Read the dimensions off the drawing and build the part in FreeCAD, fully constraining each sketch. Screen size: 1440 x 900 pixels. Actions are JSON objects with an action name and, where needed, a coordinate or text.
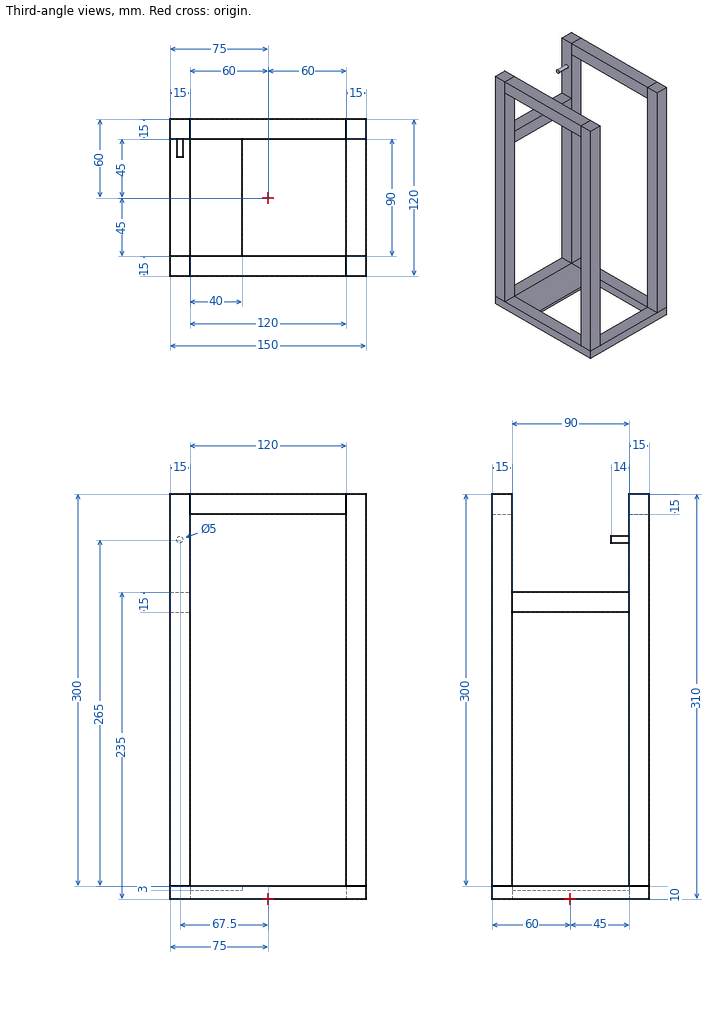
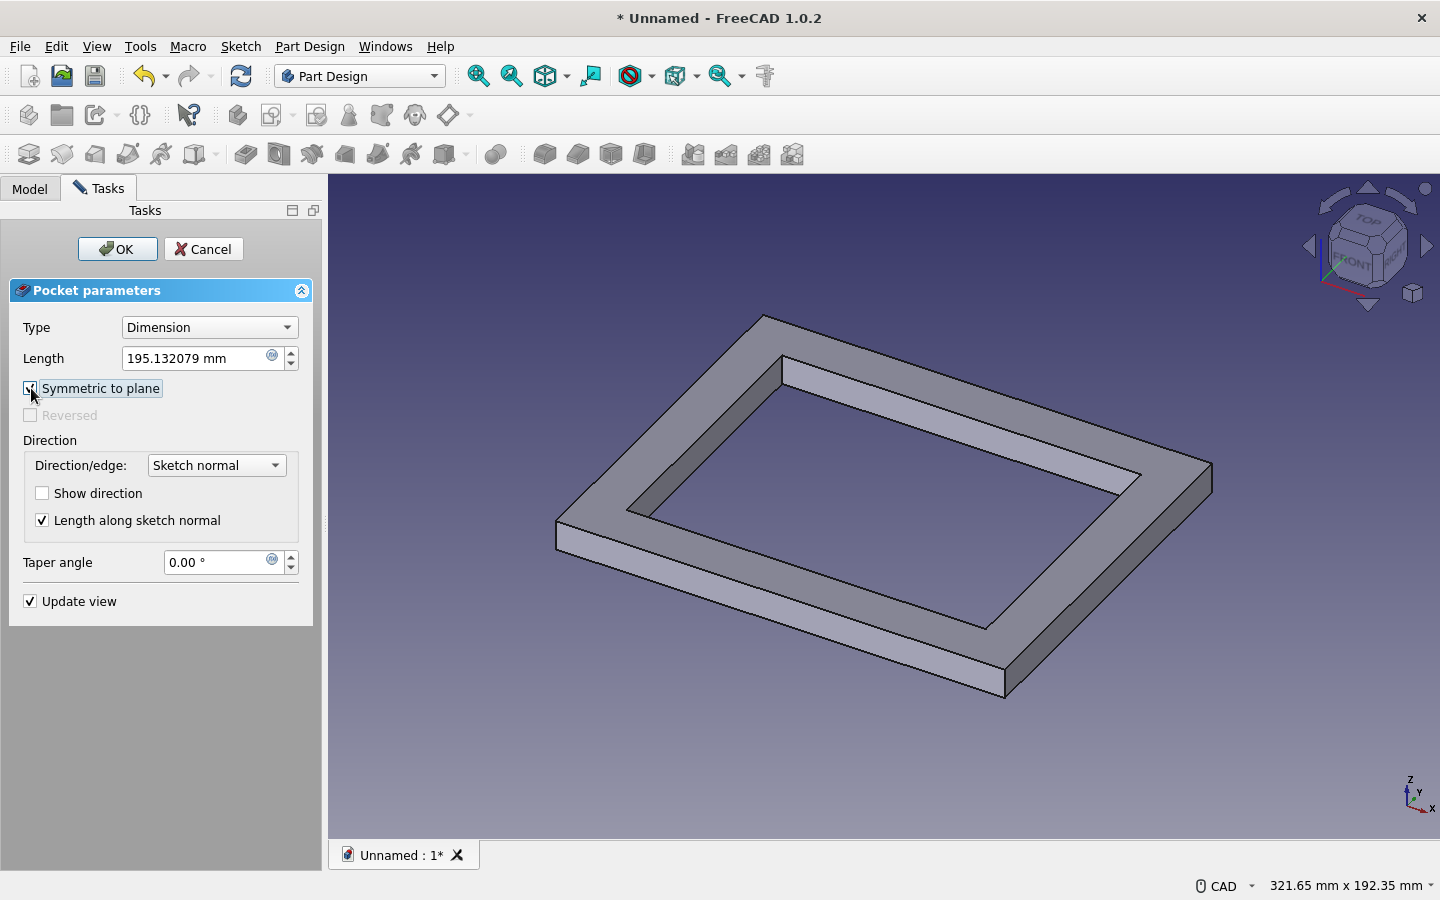
{"action": "left_click", "coordinate": [118, 249]}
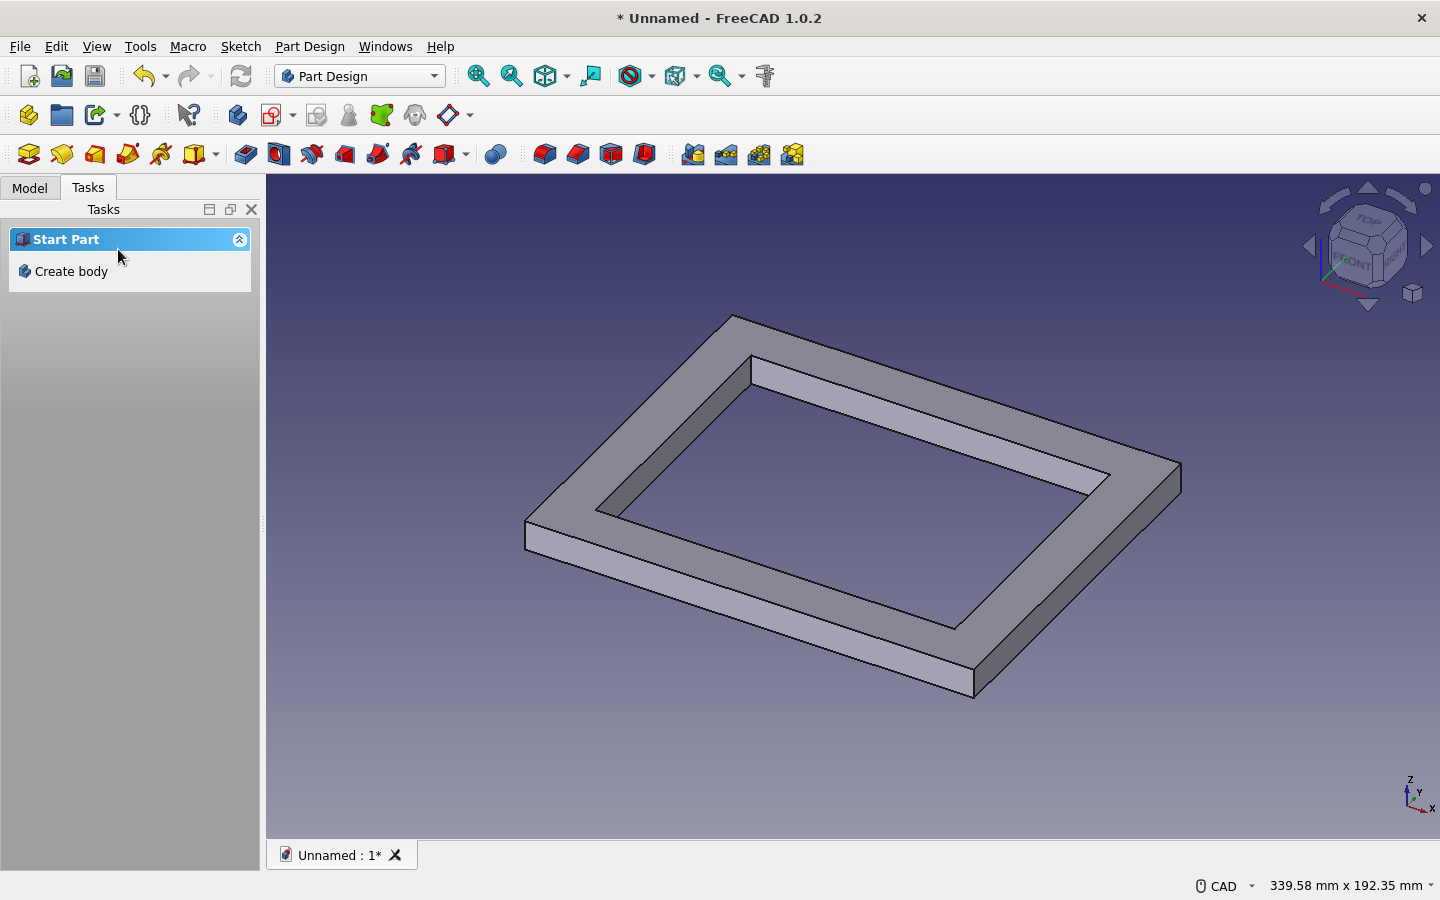
{"action": "left_click", "coordinate": [238, 116]}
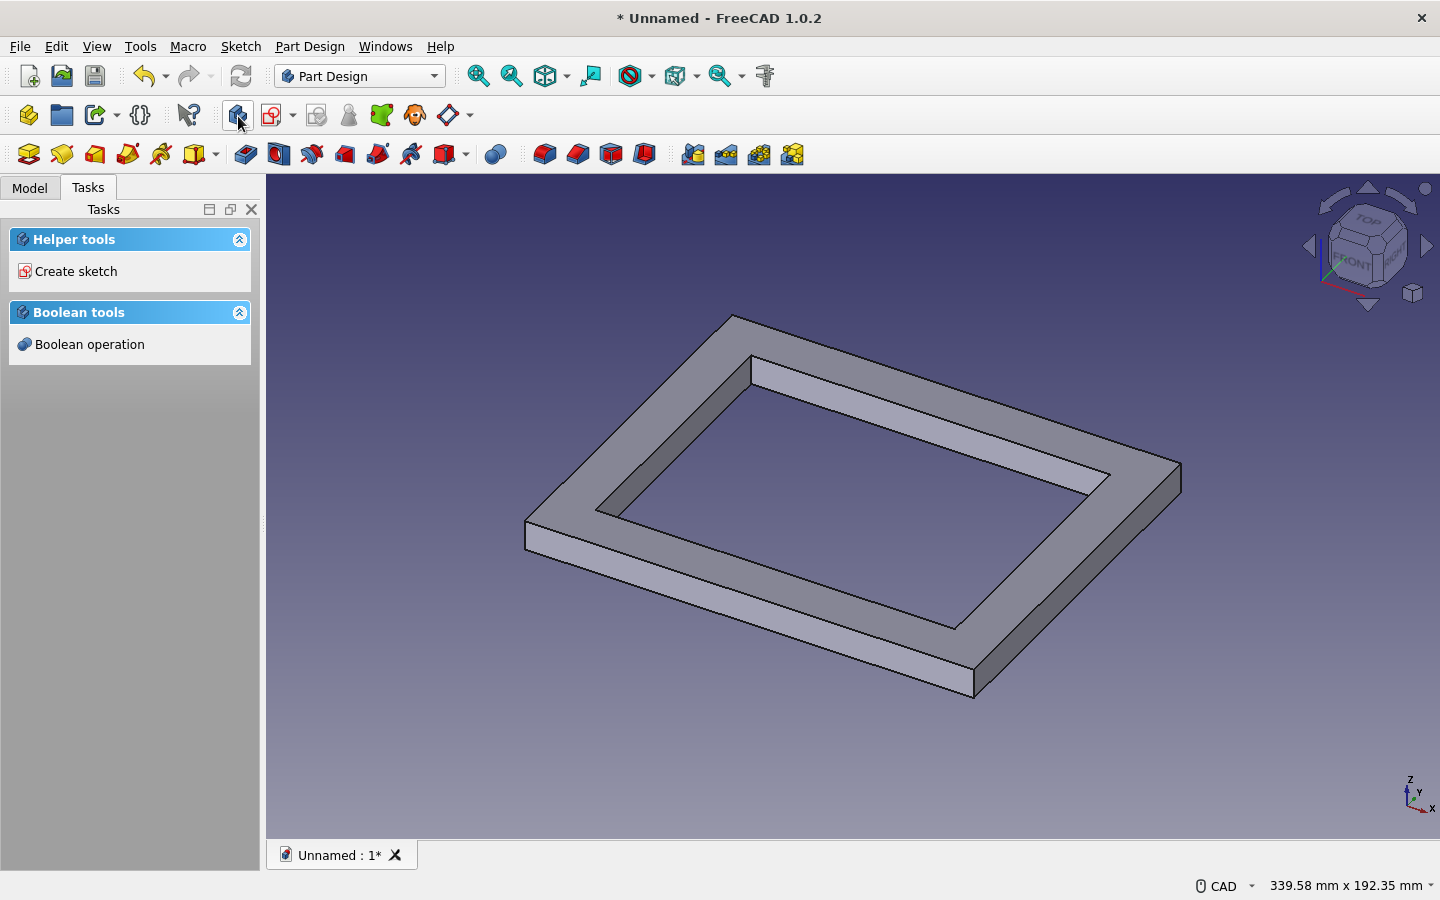
{"action": "left_click", "coordinate": [30, 188]}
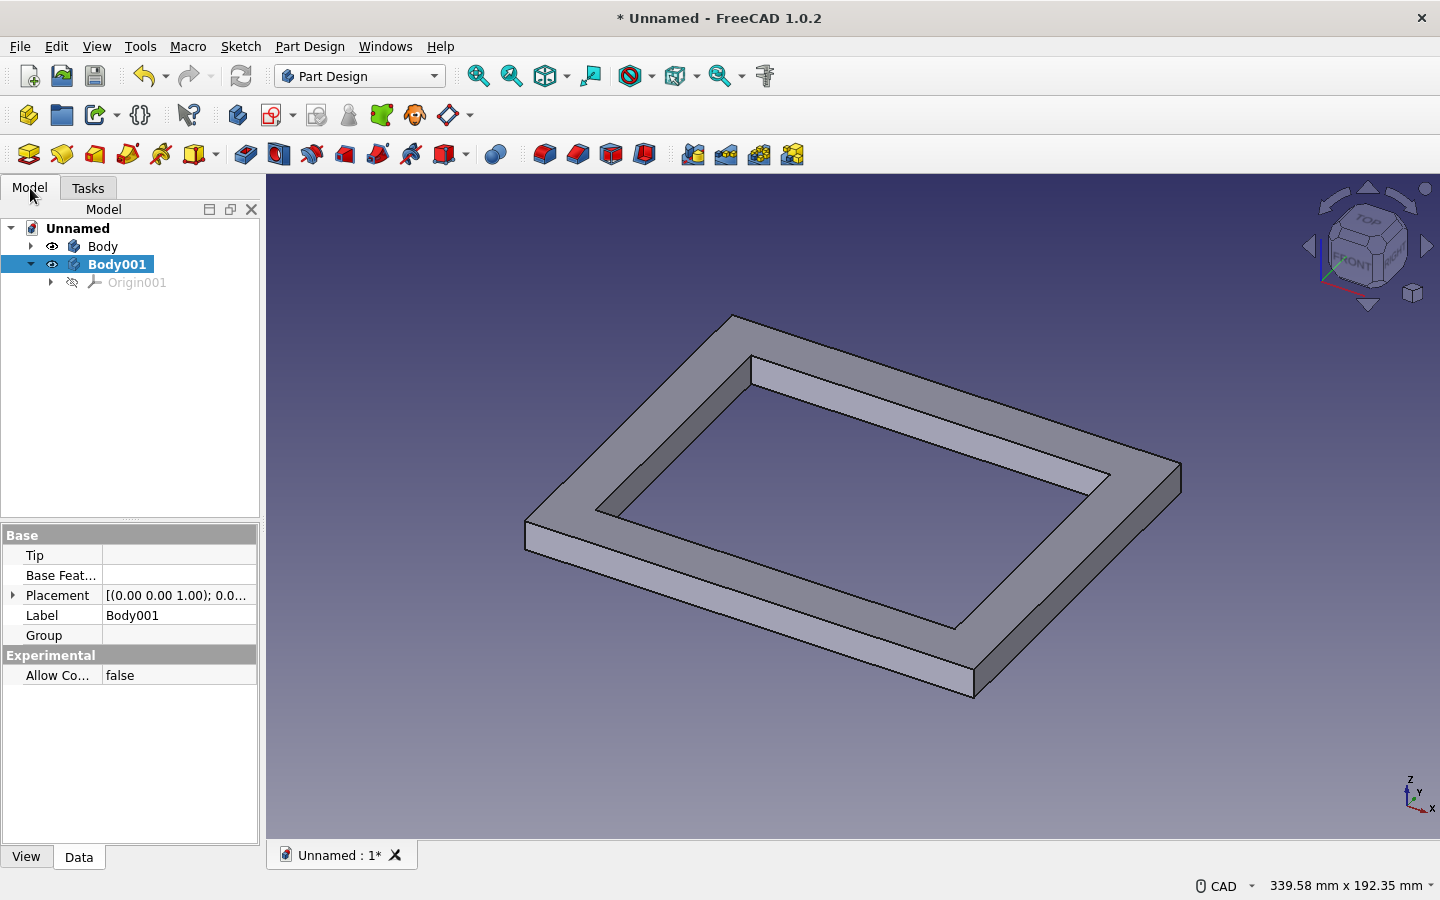
{"action": "left_click", "coordinate": [51, 282]}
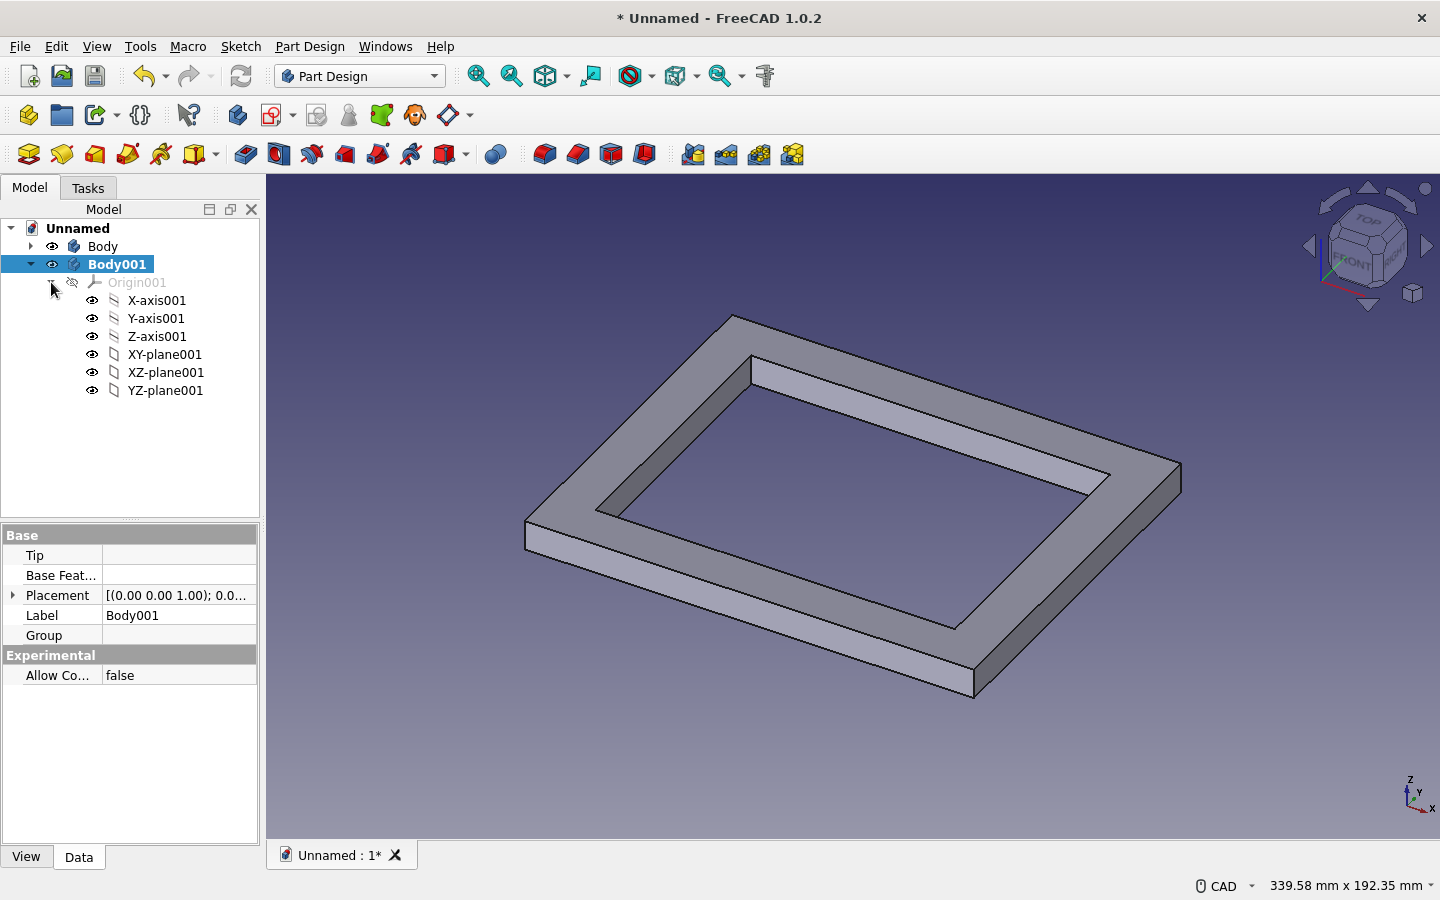
{"action": "left_click", "coordinate": [137, 354]}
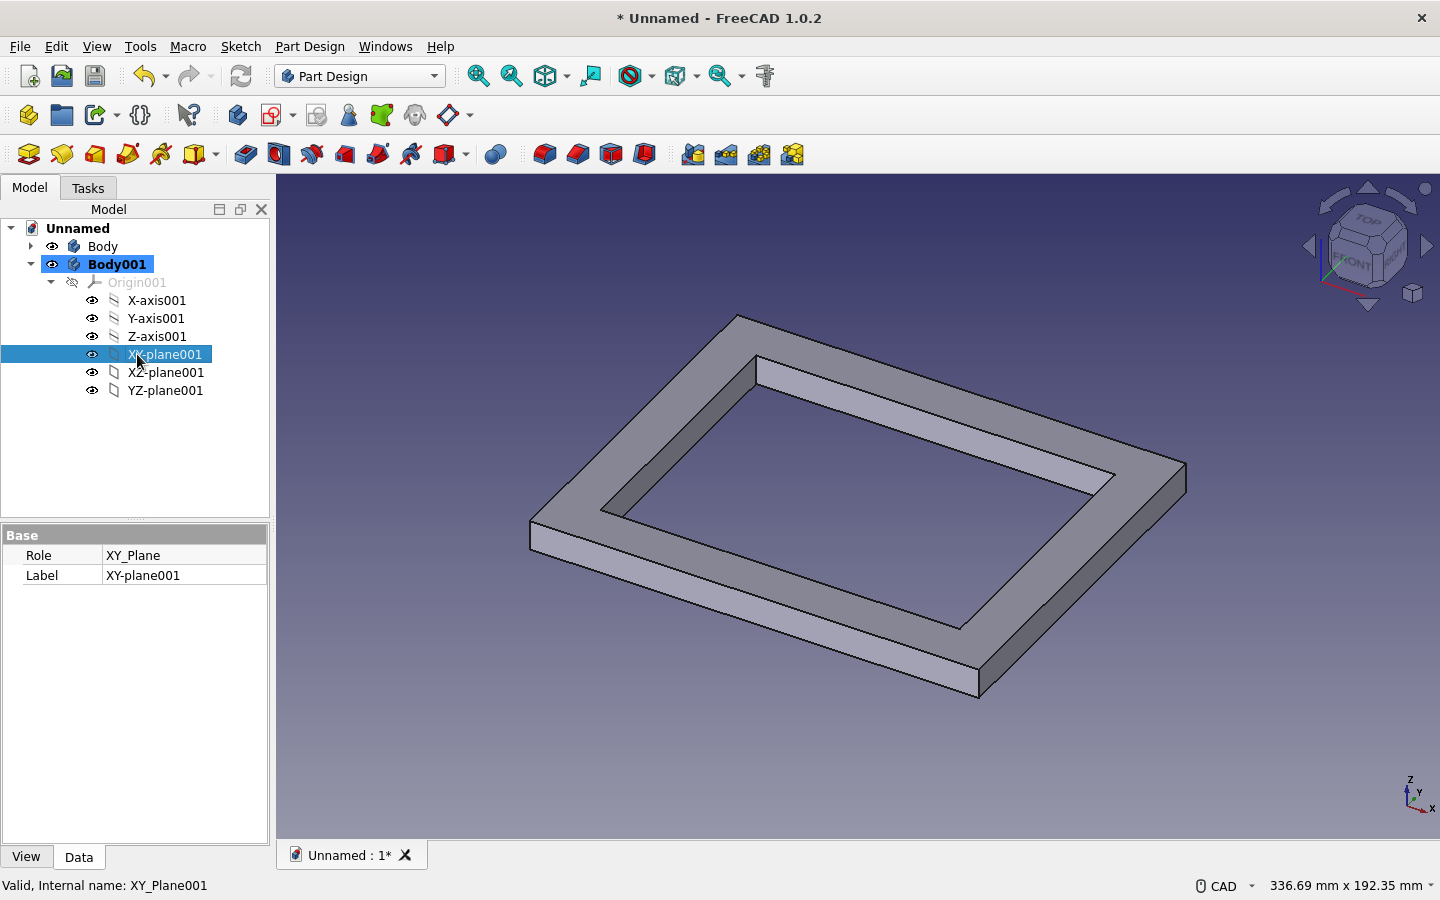
{"action": "left_click", "coordinate": [448, 116]}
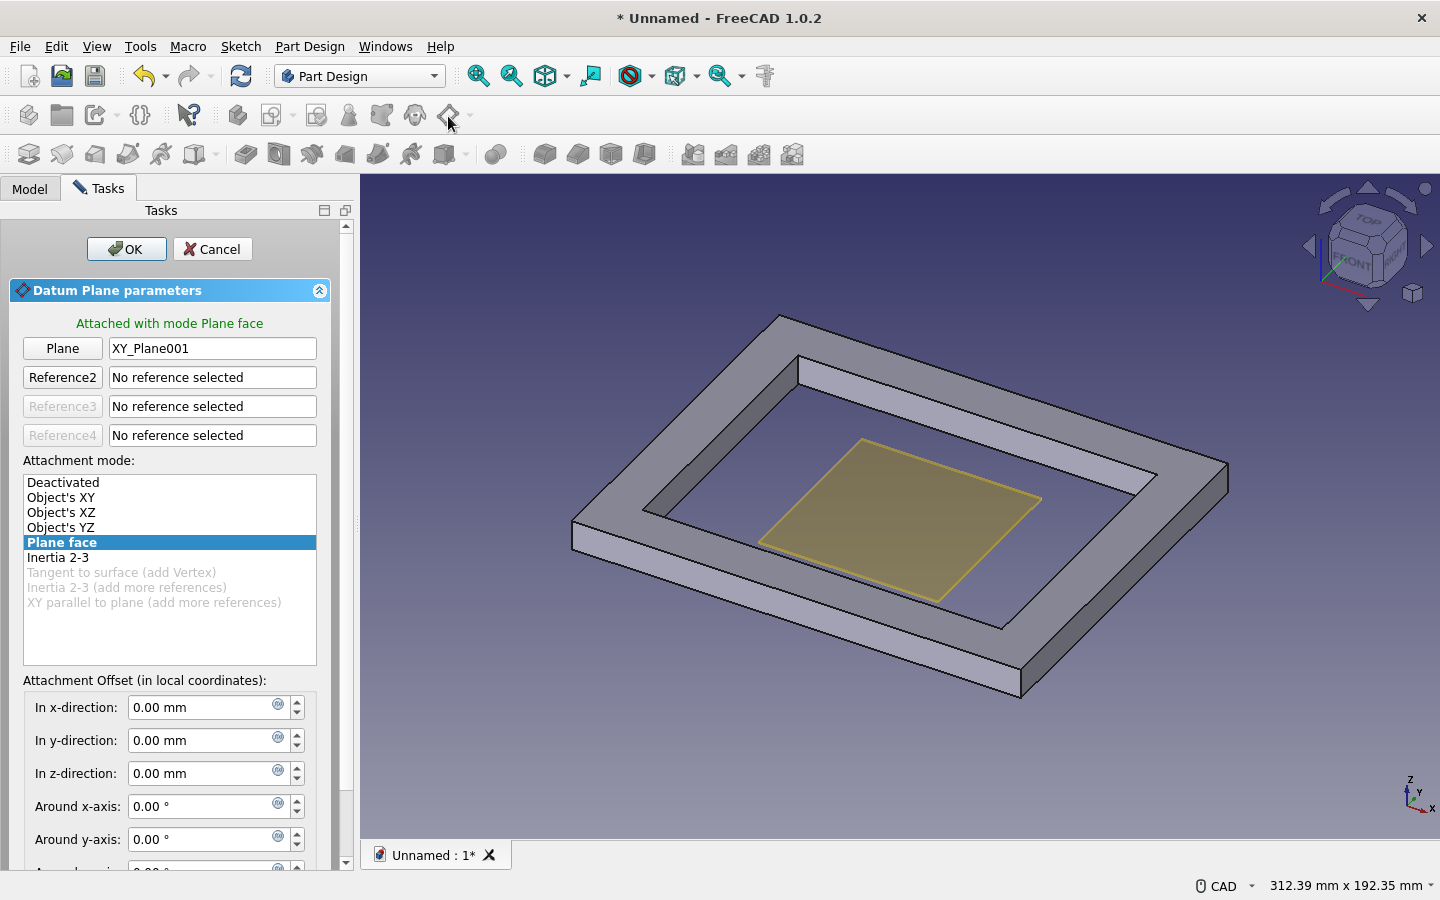
{"action": "triple_click", "coordinate": [210, 774]}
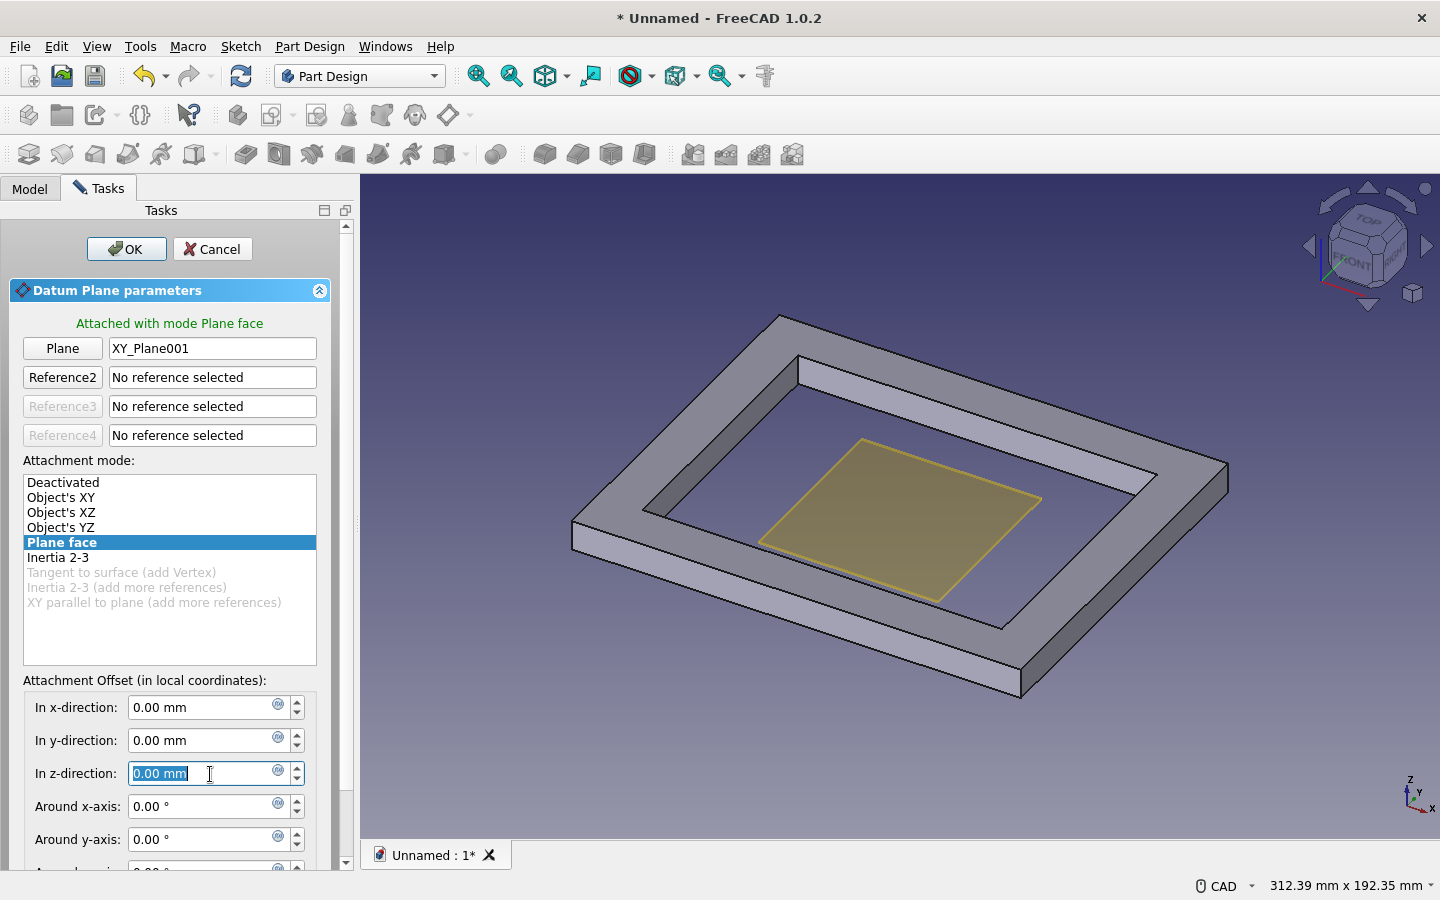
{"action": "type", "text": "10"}
{"action": "key", "text": "Tab"}